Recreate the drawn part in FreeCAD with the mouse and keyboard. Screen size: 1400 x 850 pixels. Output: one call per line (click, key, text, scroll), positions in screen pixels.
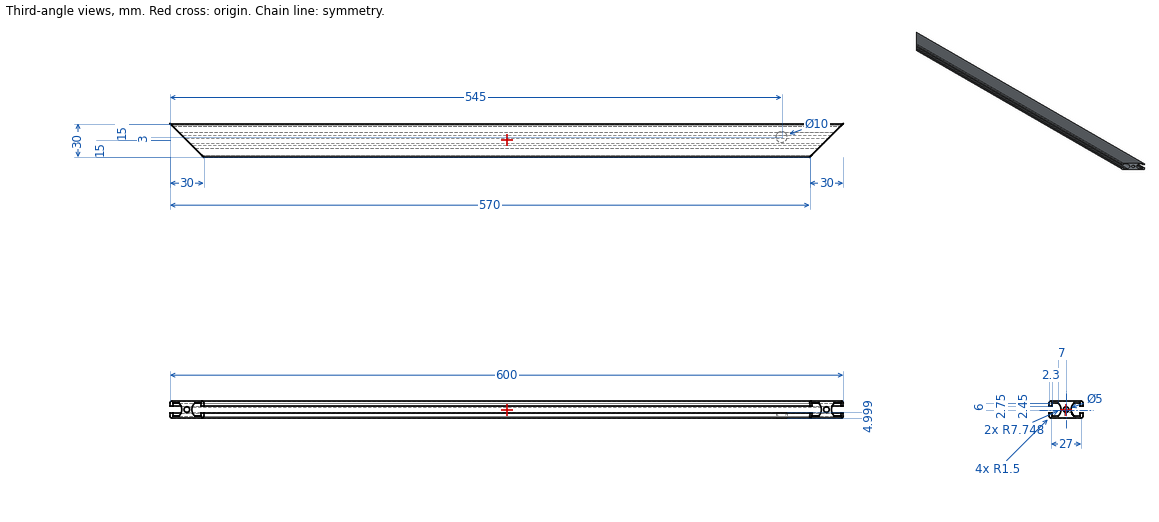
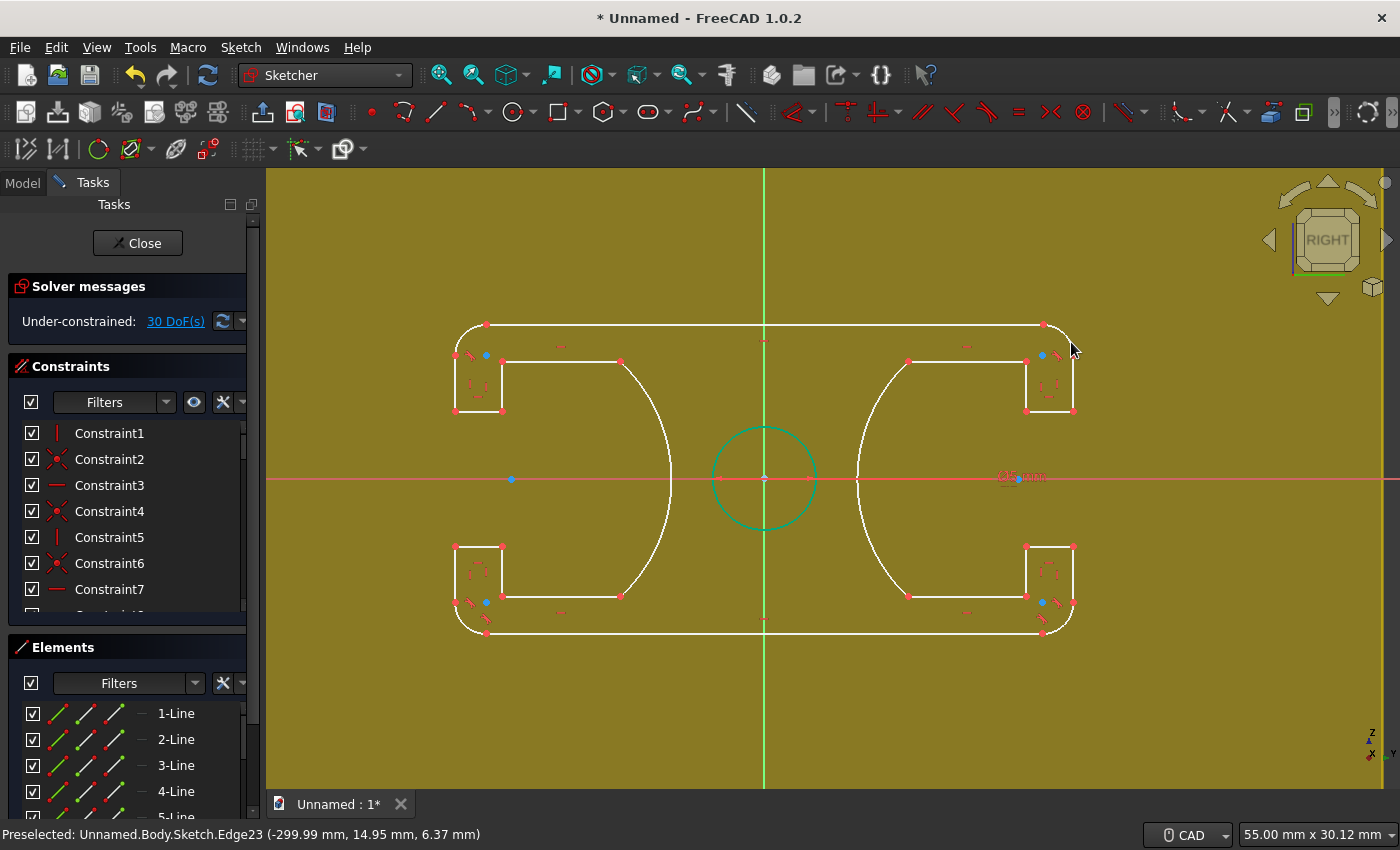
click(876, 325)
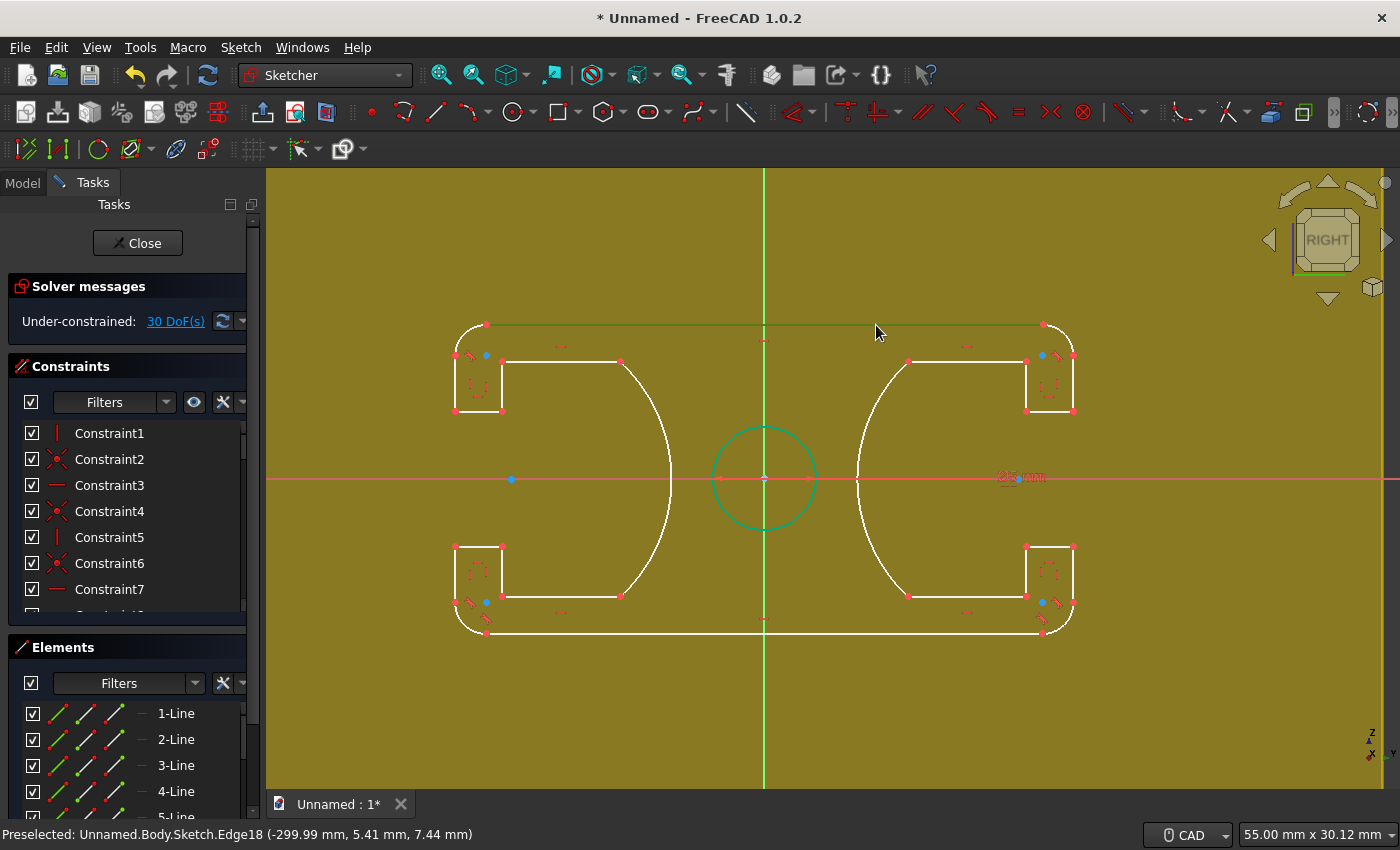
click(1070, 342)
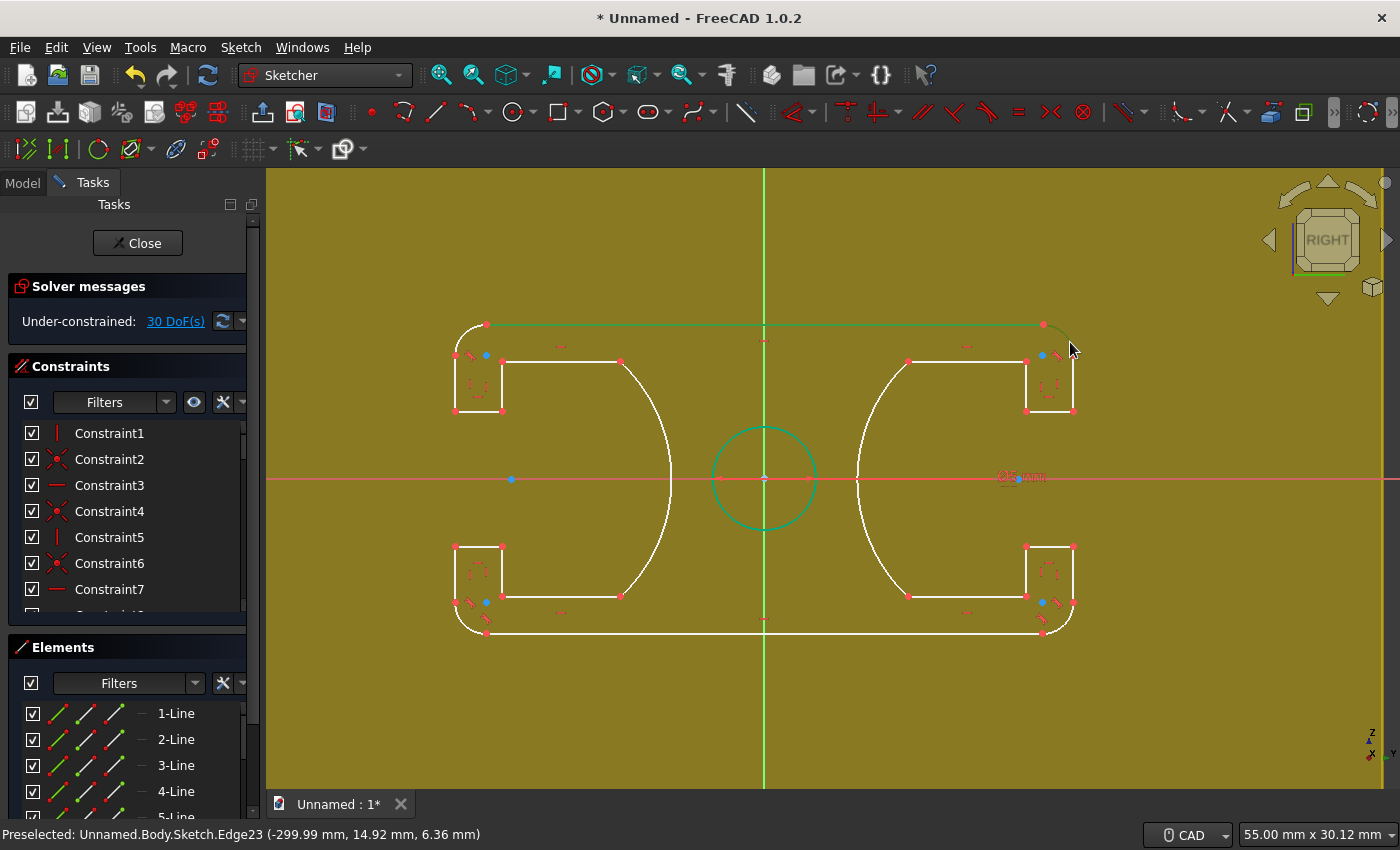
click(988, 112)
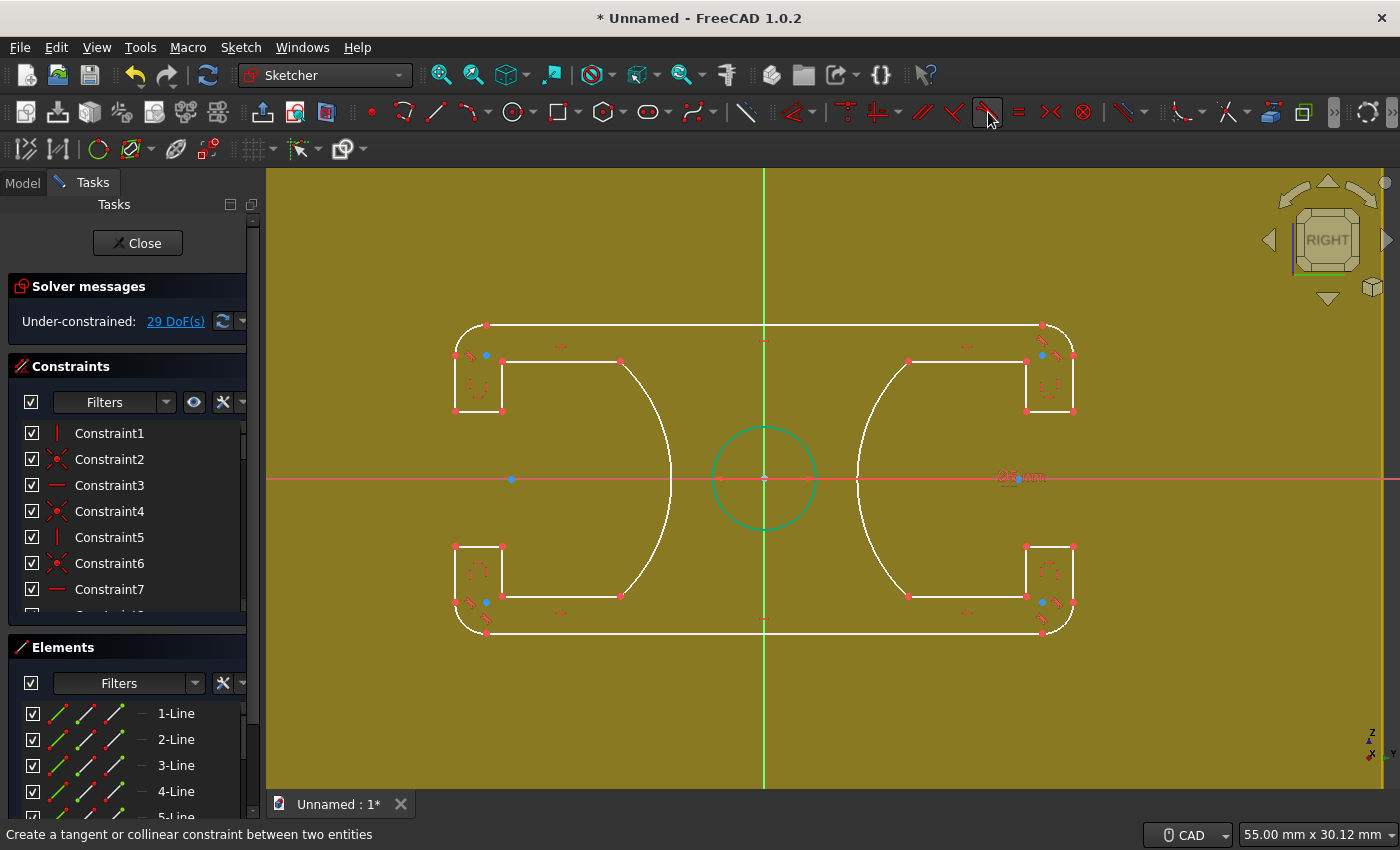
click(876, 325)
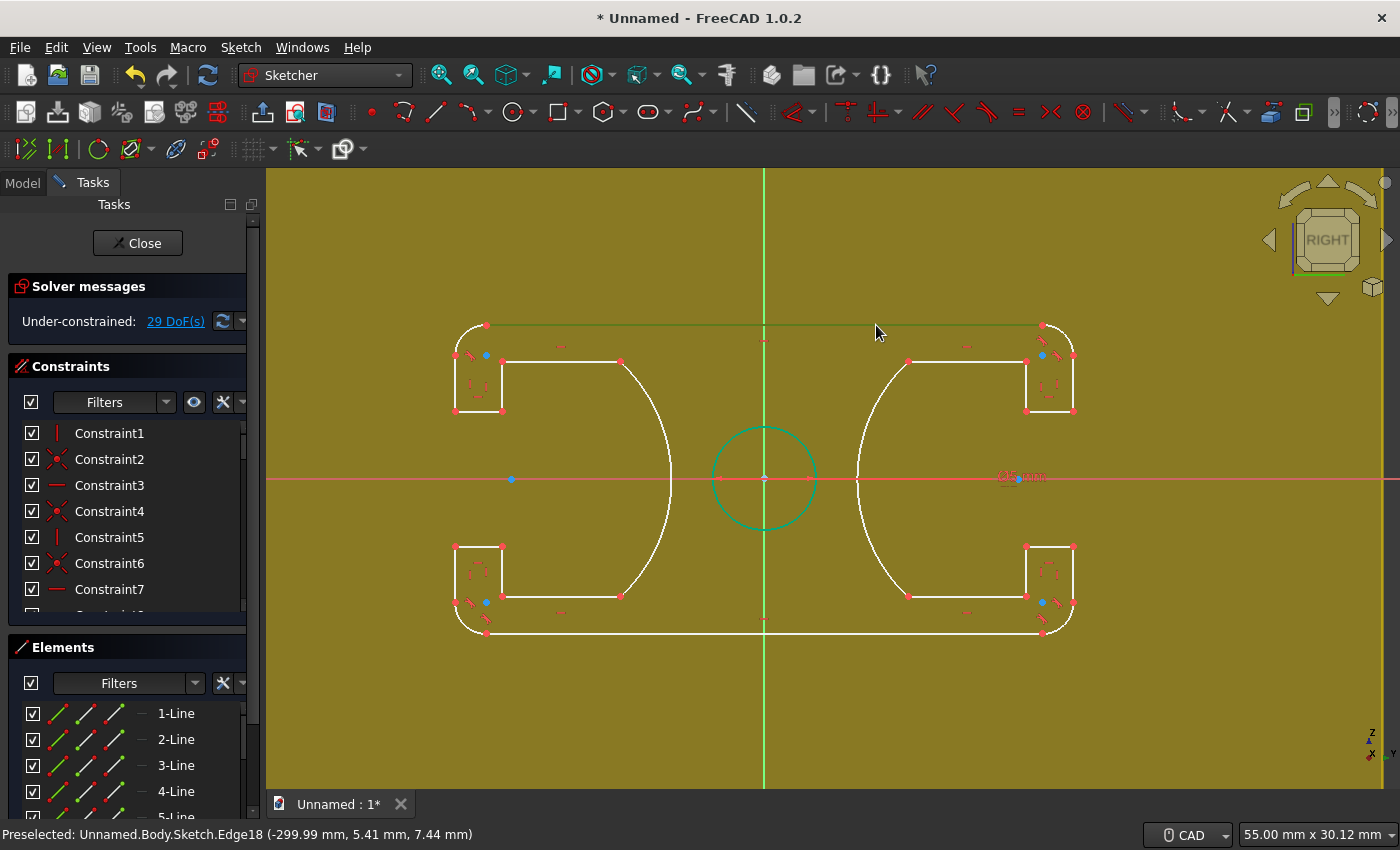
click(472, 328)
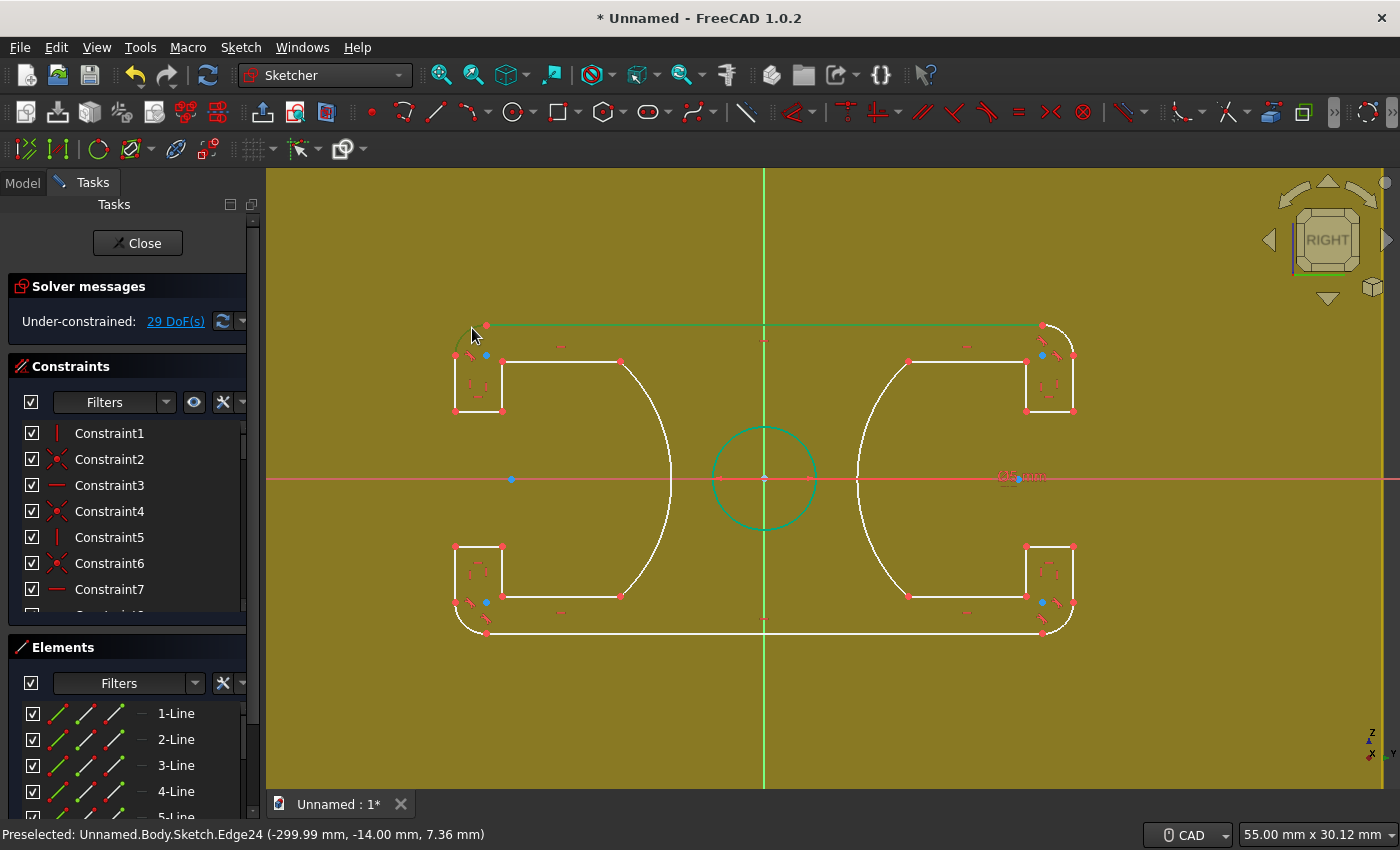
key(t)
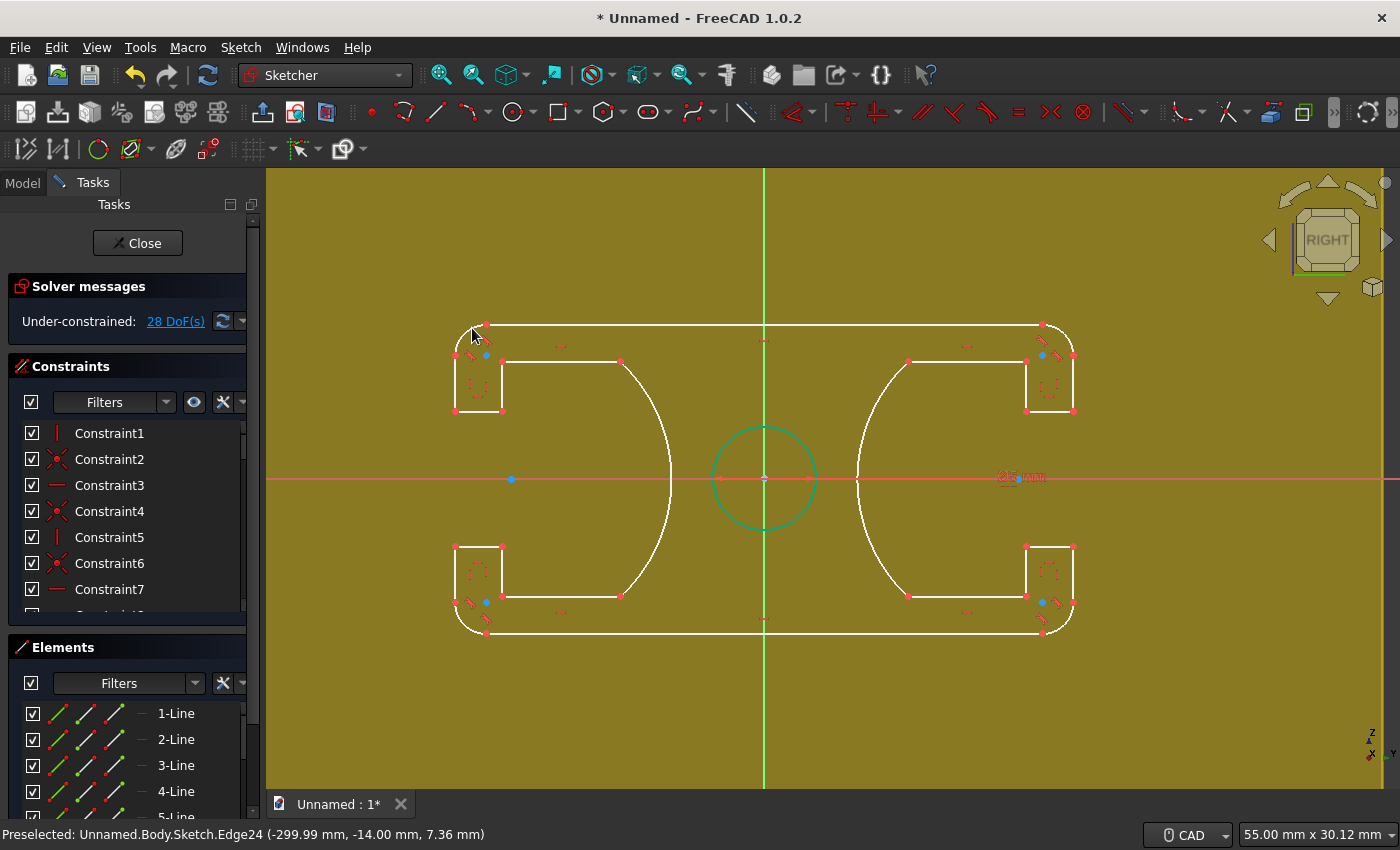
click(459, 617)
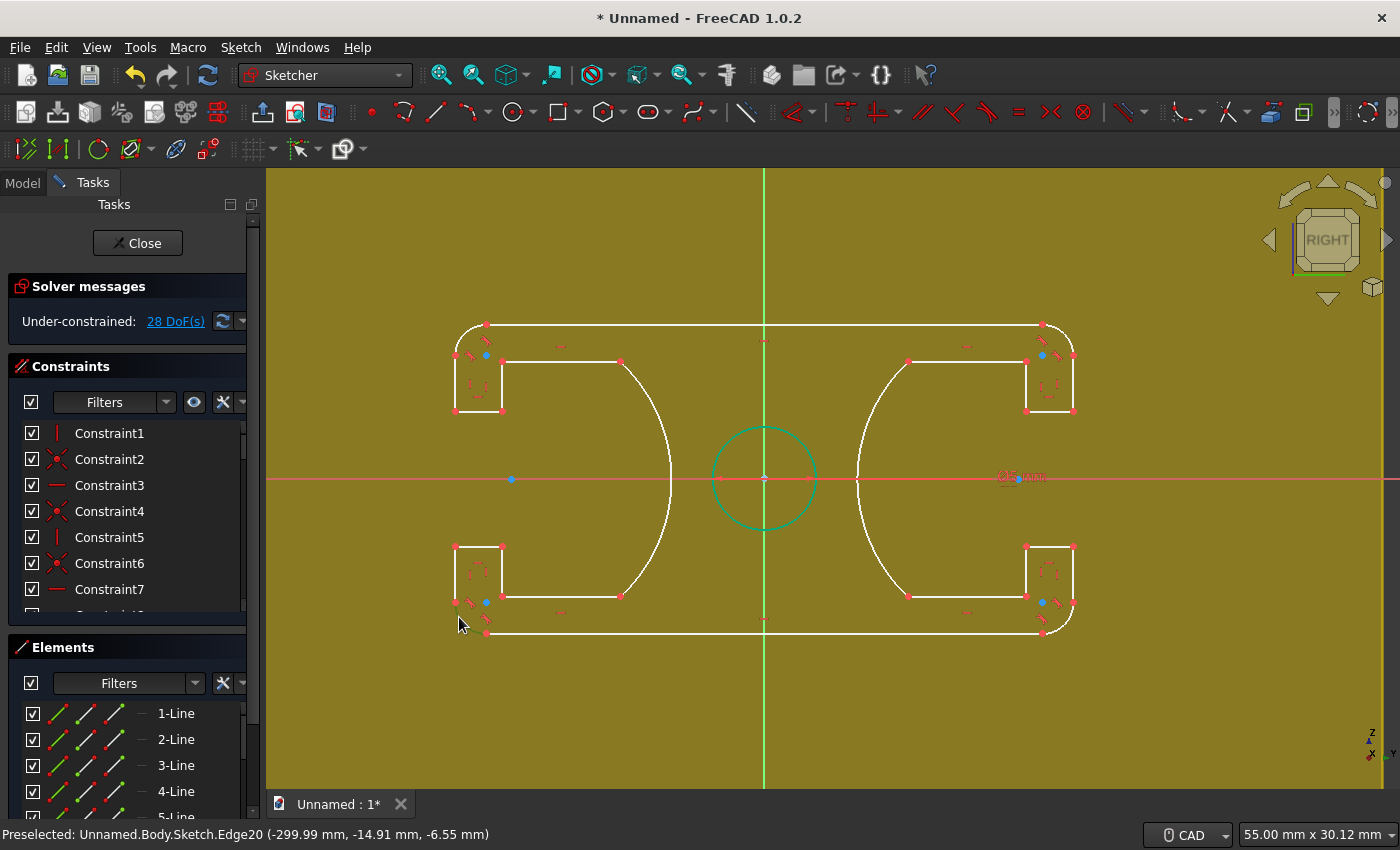
click(1056, 631)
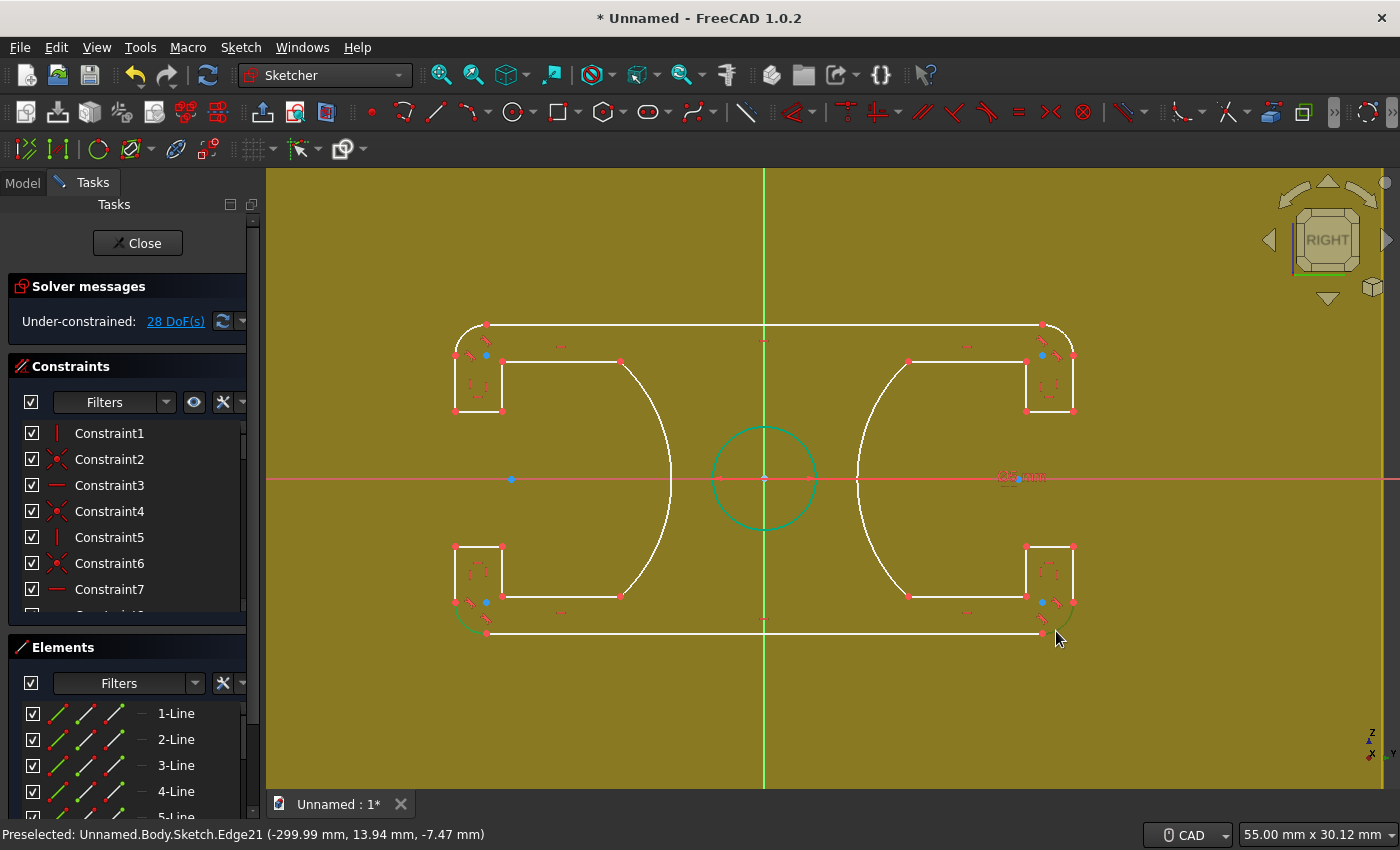
click(1070, 342)